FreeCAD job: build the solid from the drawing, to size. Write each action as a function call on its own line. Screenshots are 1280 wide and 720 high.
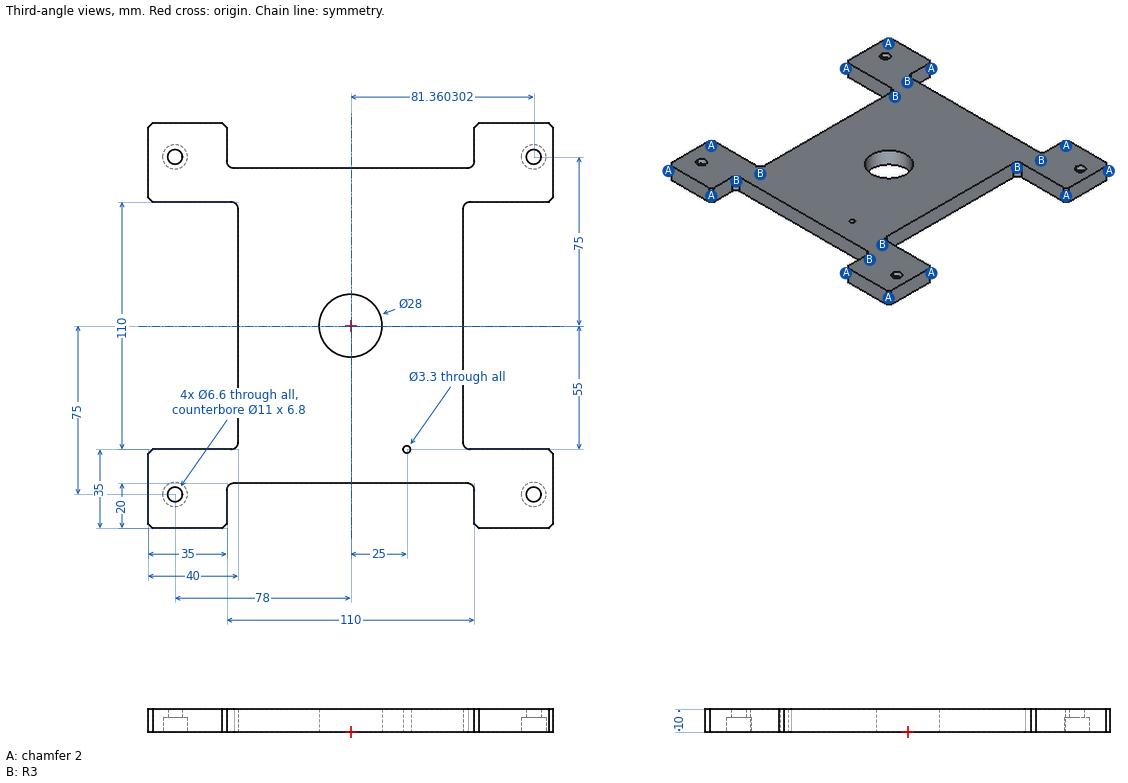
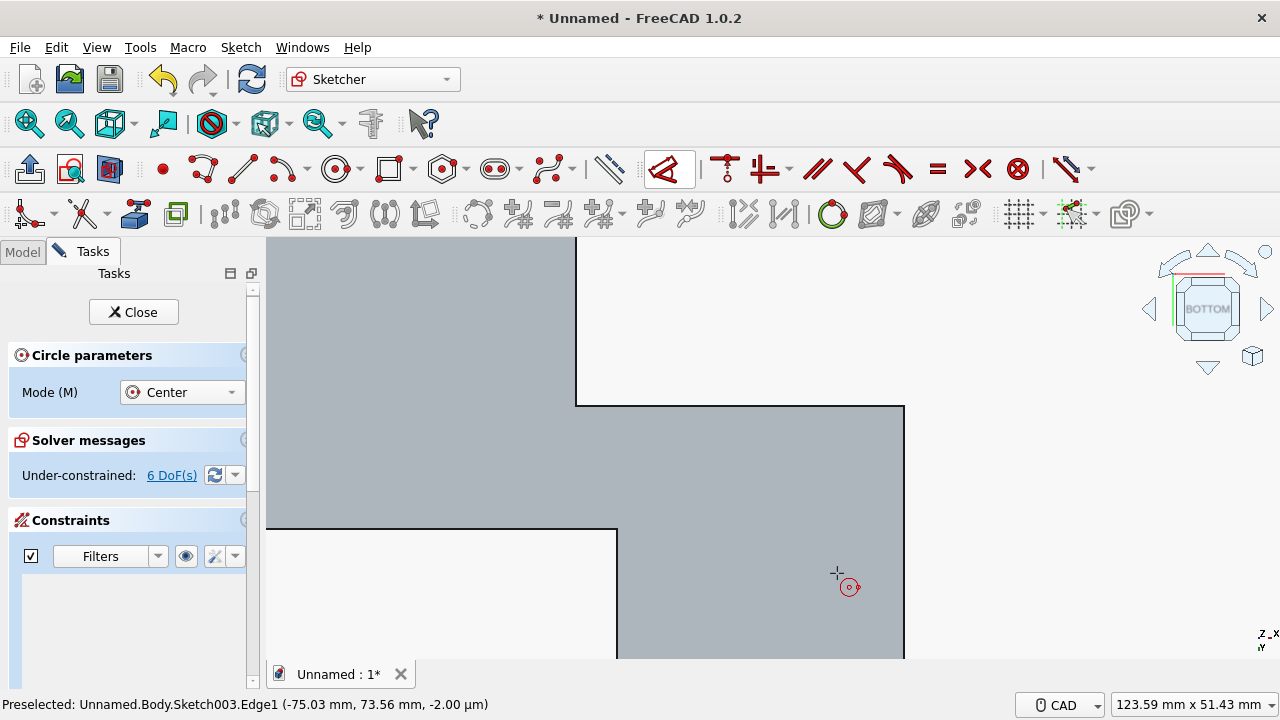
scroll(837, 573, down, 8)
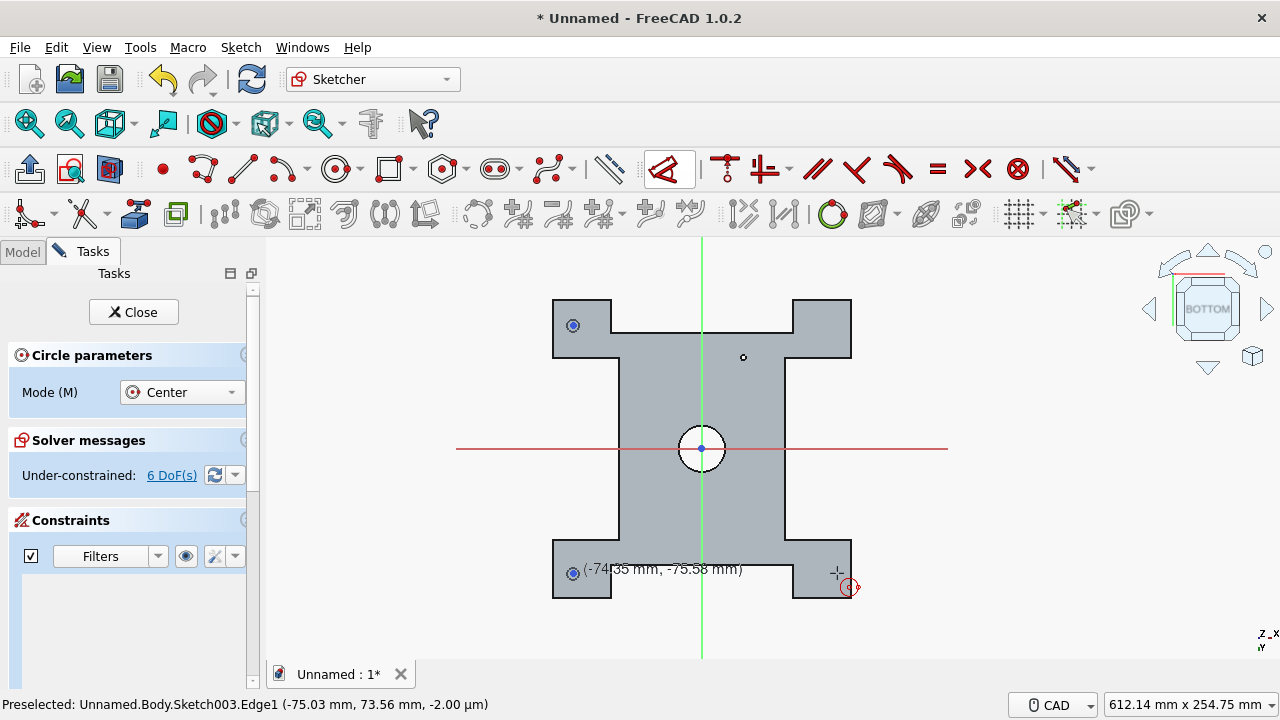
click(837, 573)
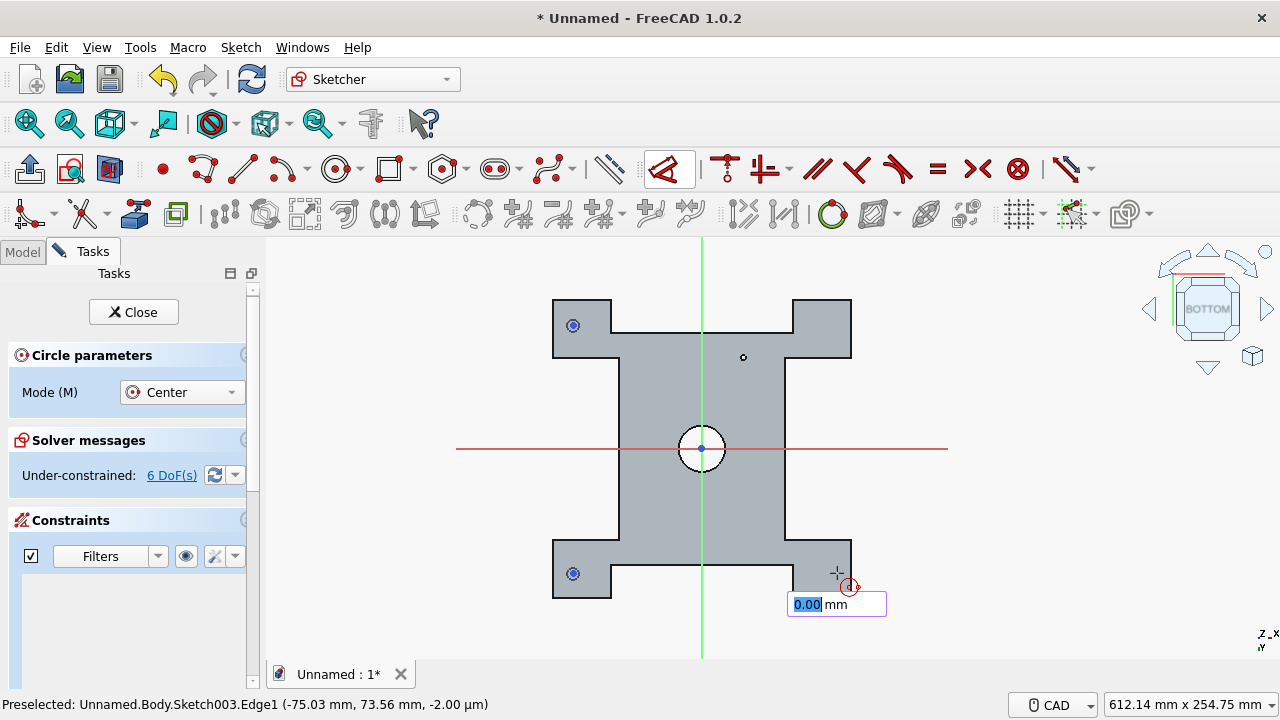
scroll(841, 569, up, 6)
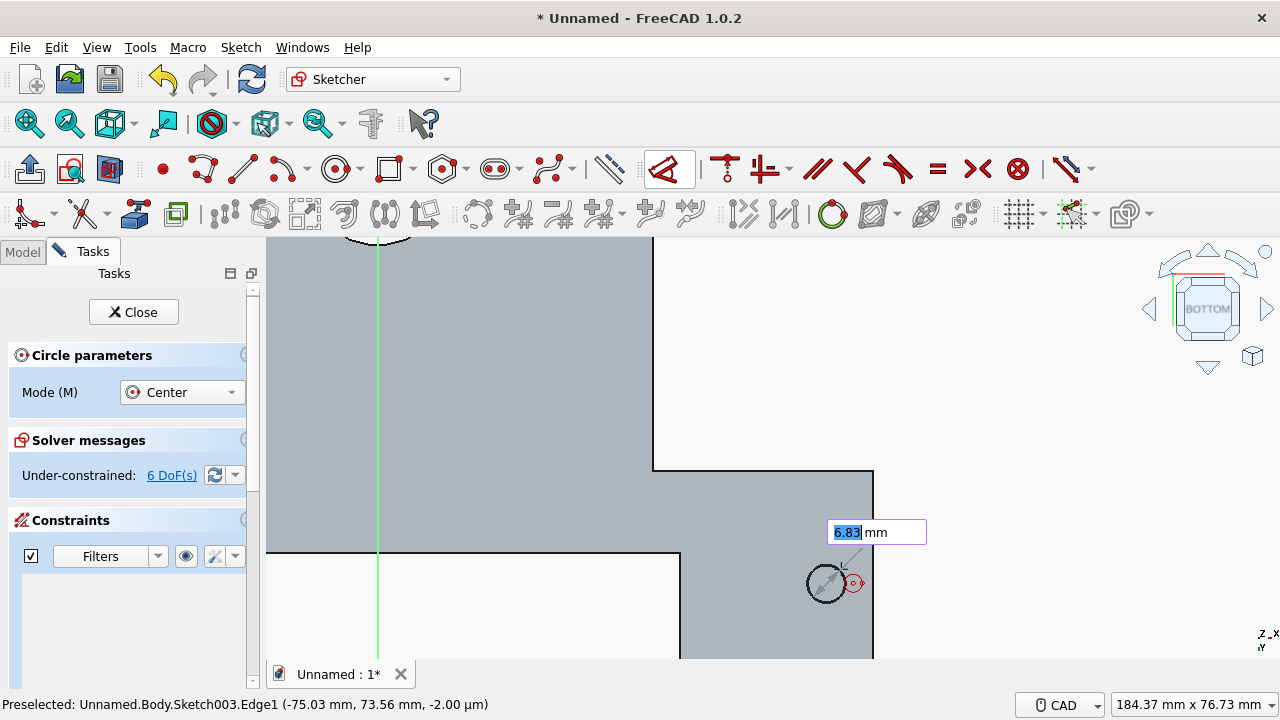
click(838, 568)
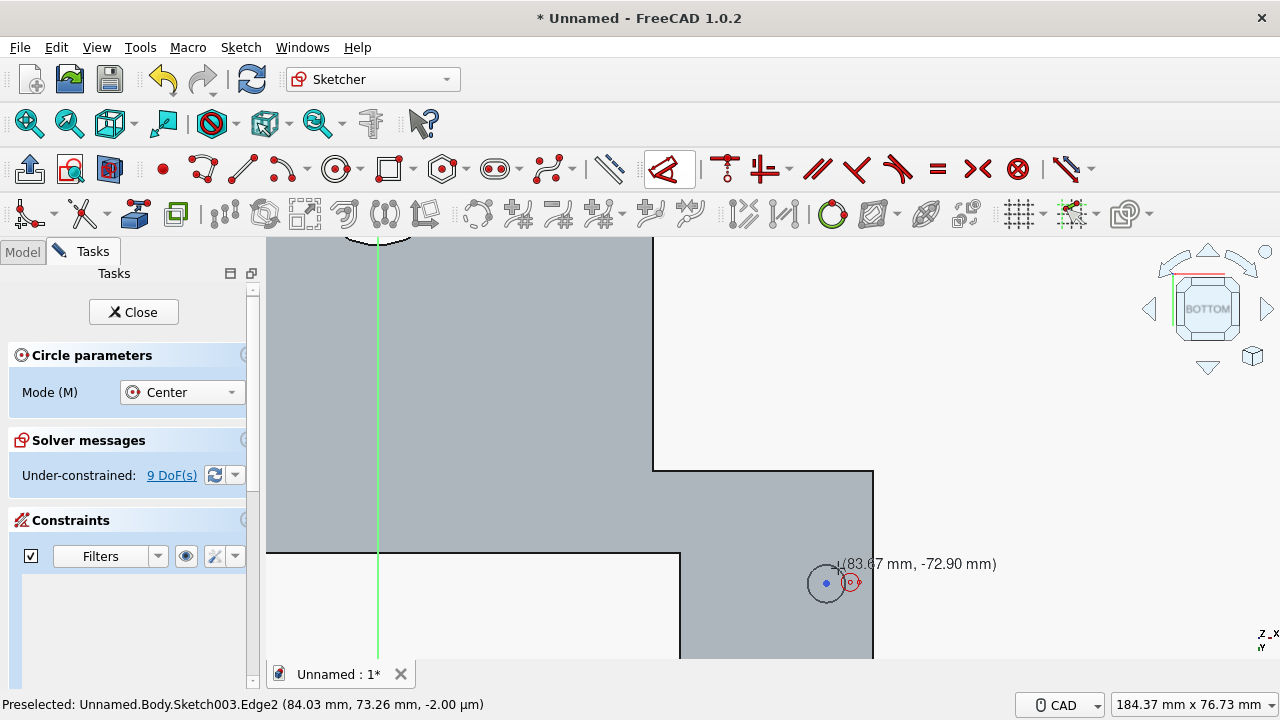
scroll(841, 569, down, 6)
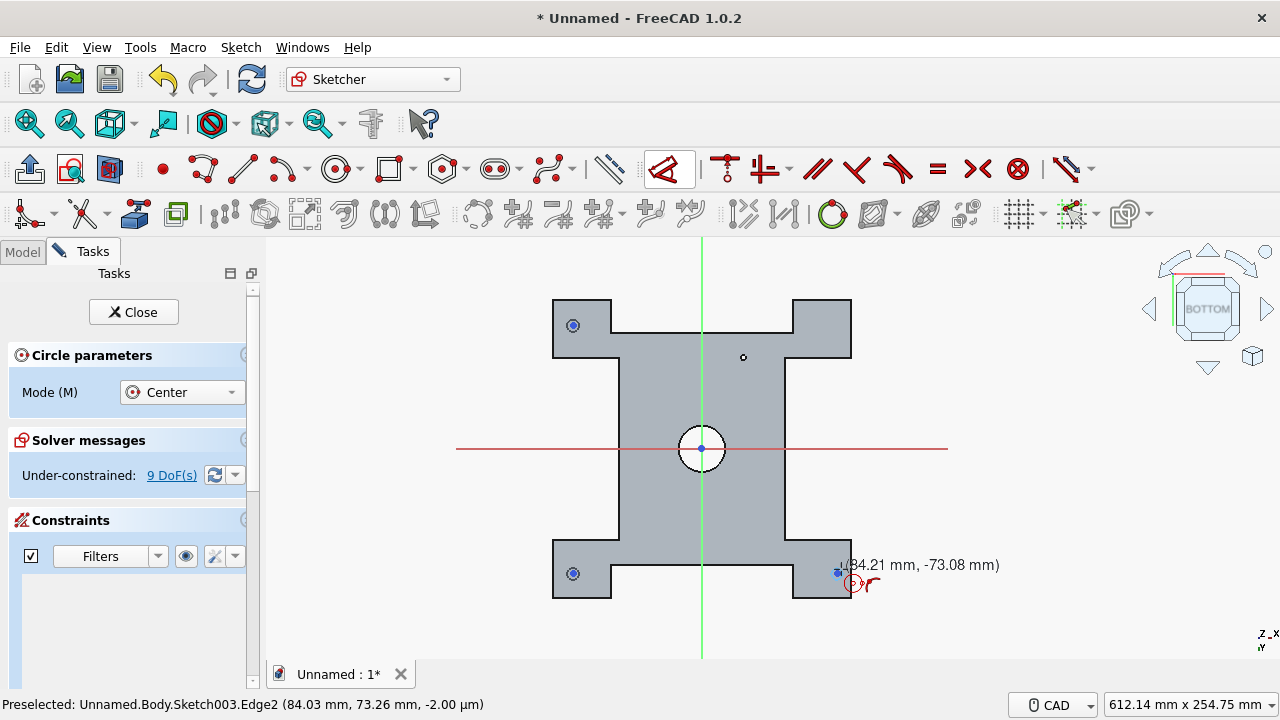
scroll(837, 325, up, 8)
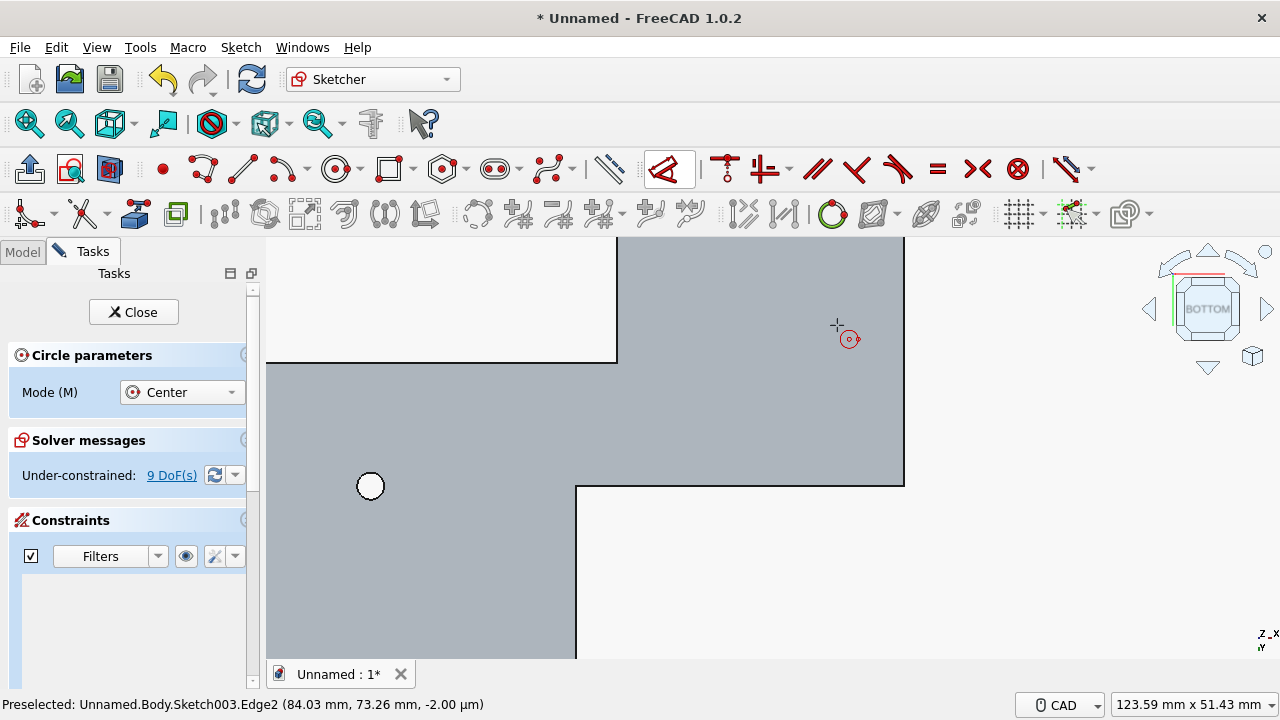
scroll(837, 324, down, 8)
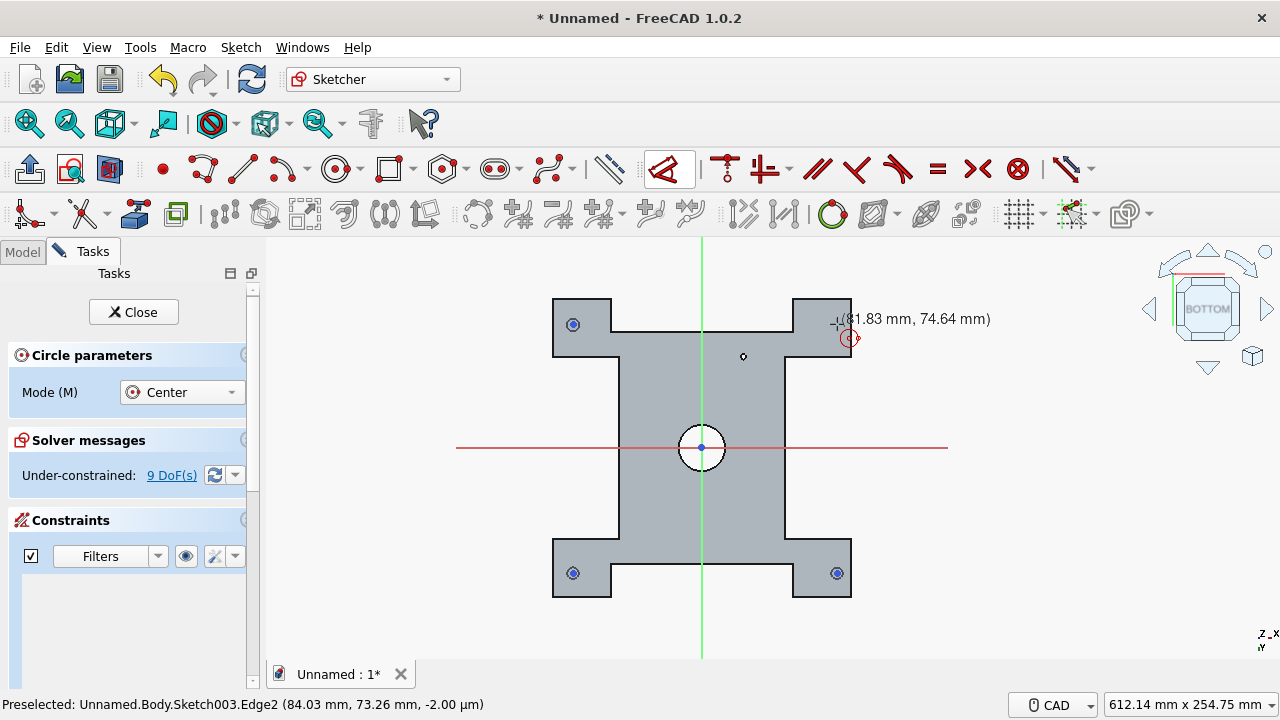
click(837, 324)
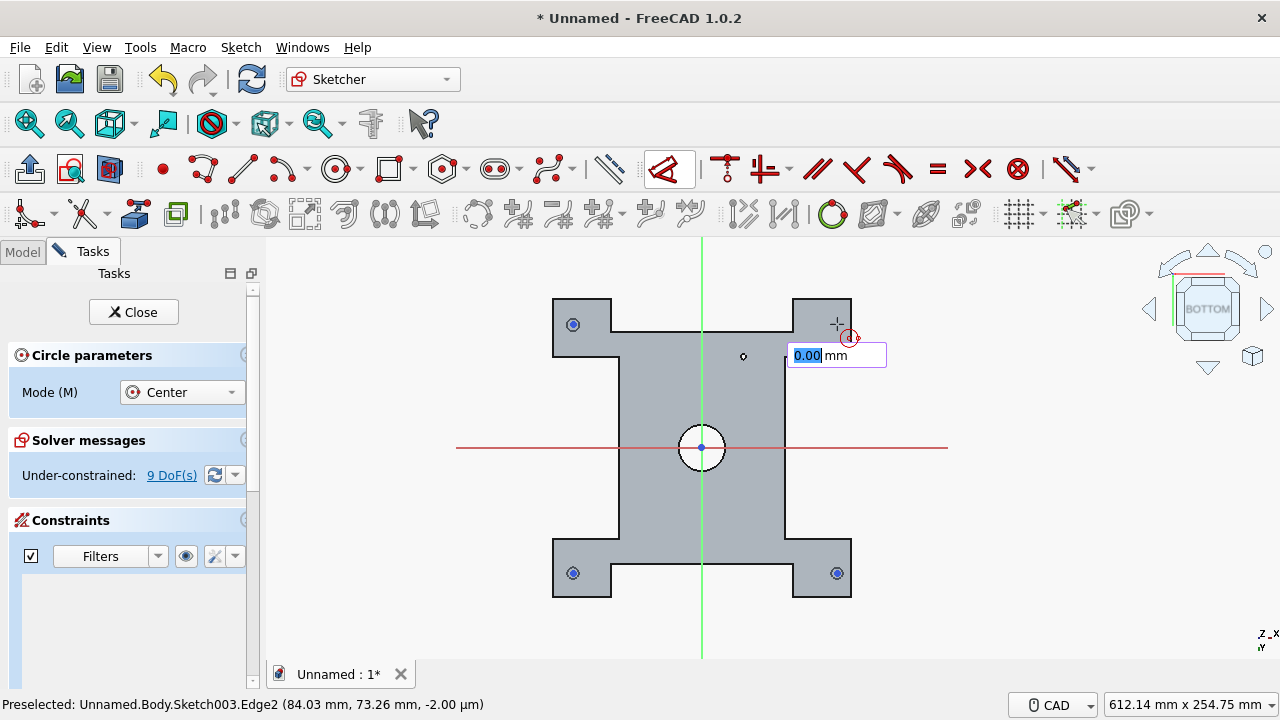
scroll(841, 320, up, 6)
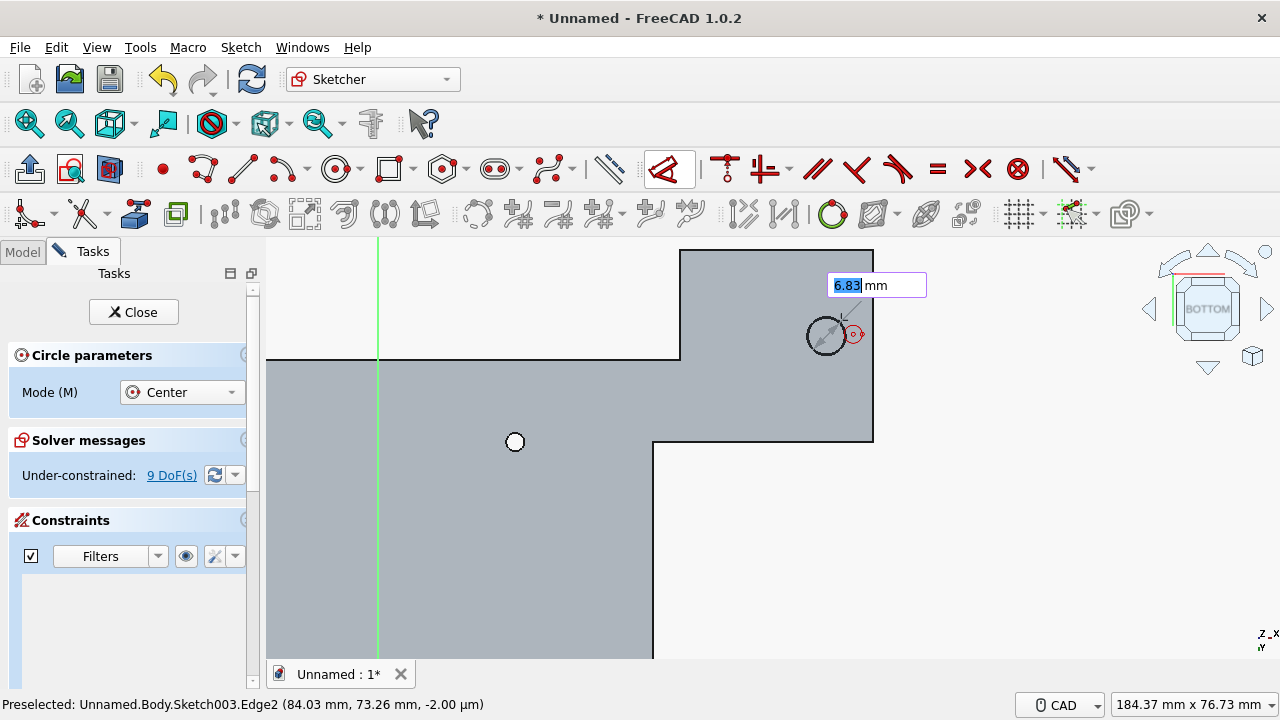
click(838, 319)
key(Escape)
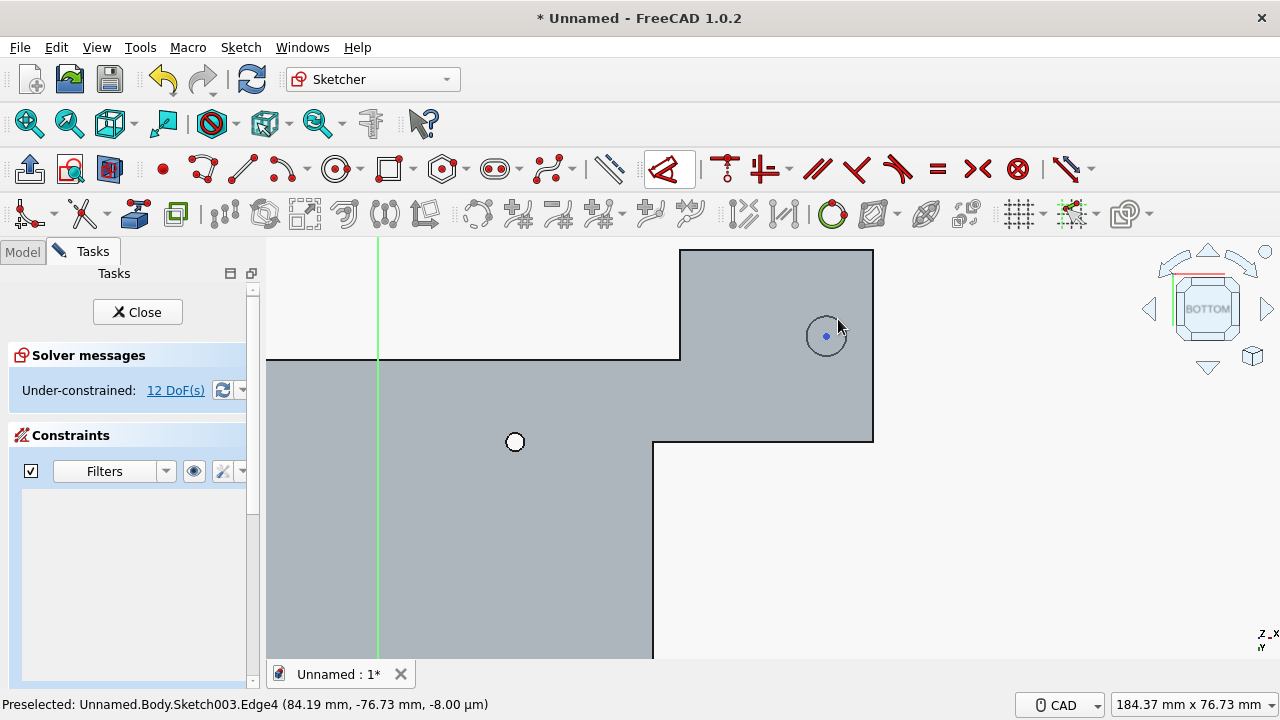
scroll(841, 320, down, 6)